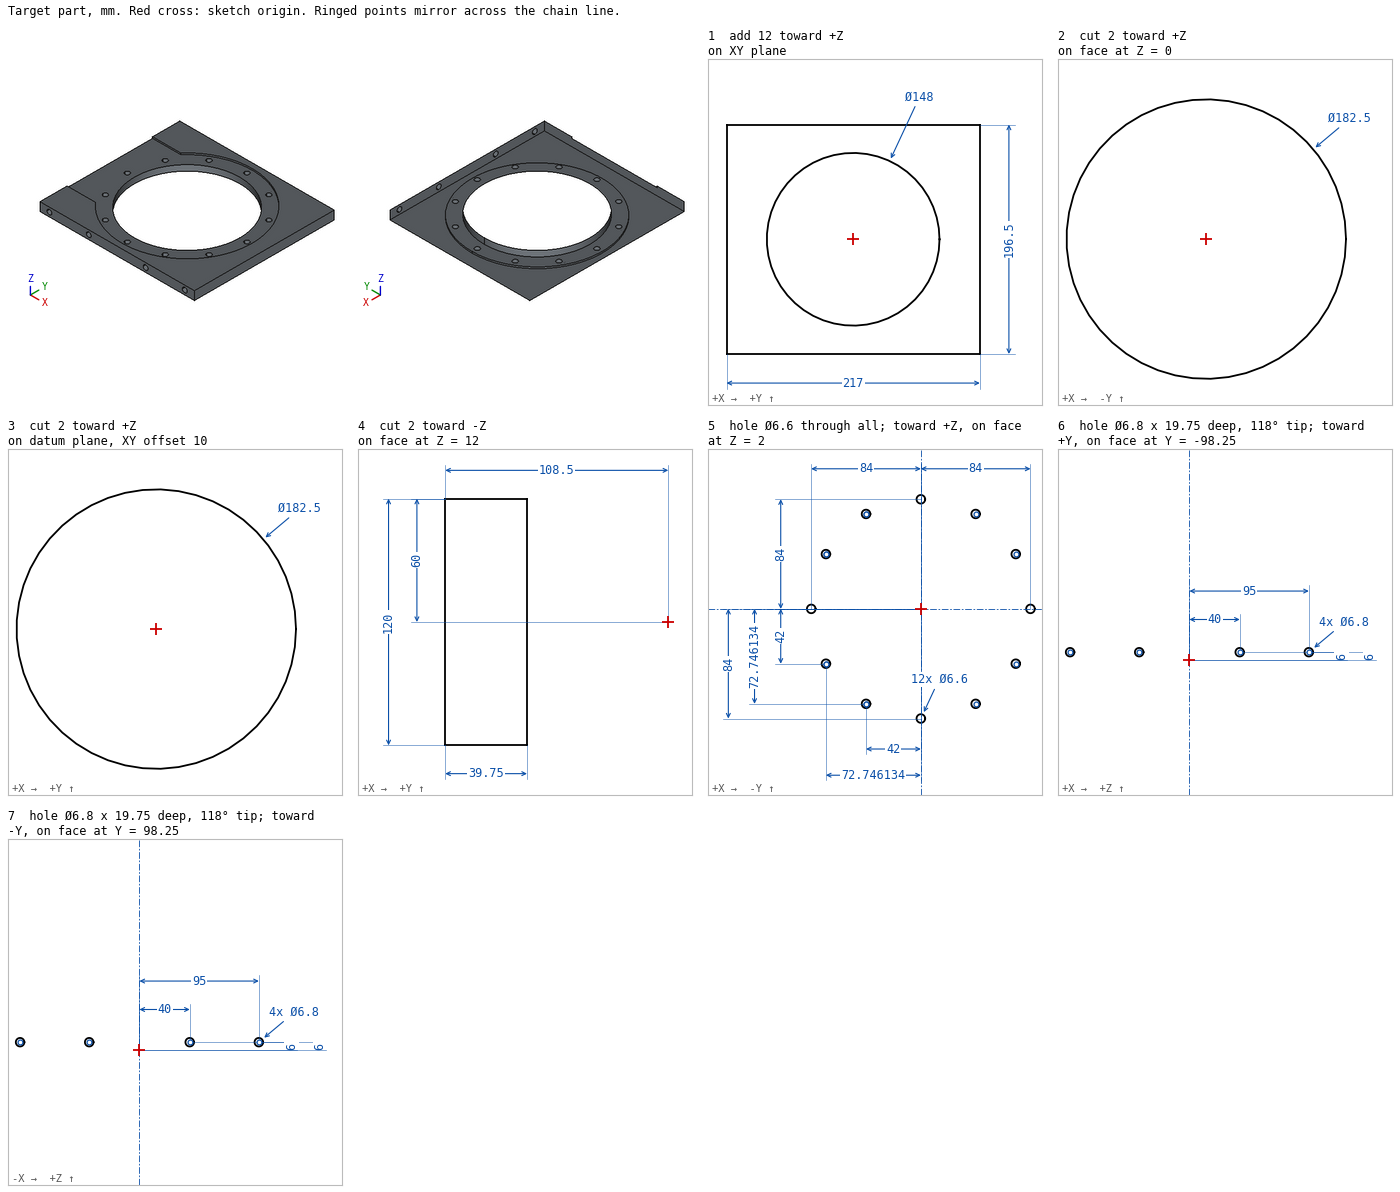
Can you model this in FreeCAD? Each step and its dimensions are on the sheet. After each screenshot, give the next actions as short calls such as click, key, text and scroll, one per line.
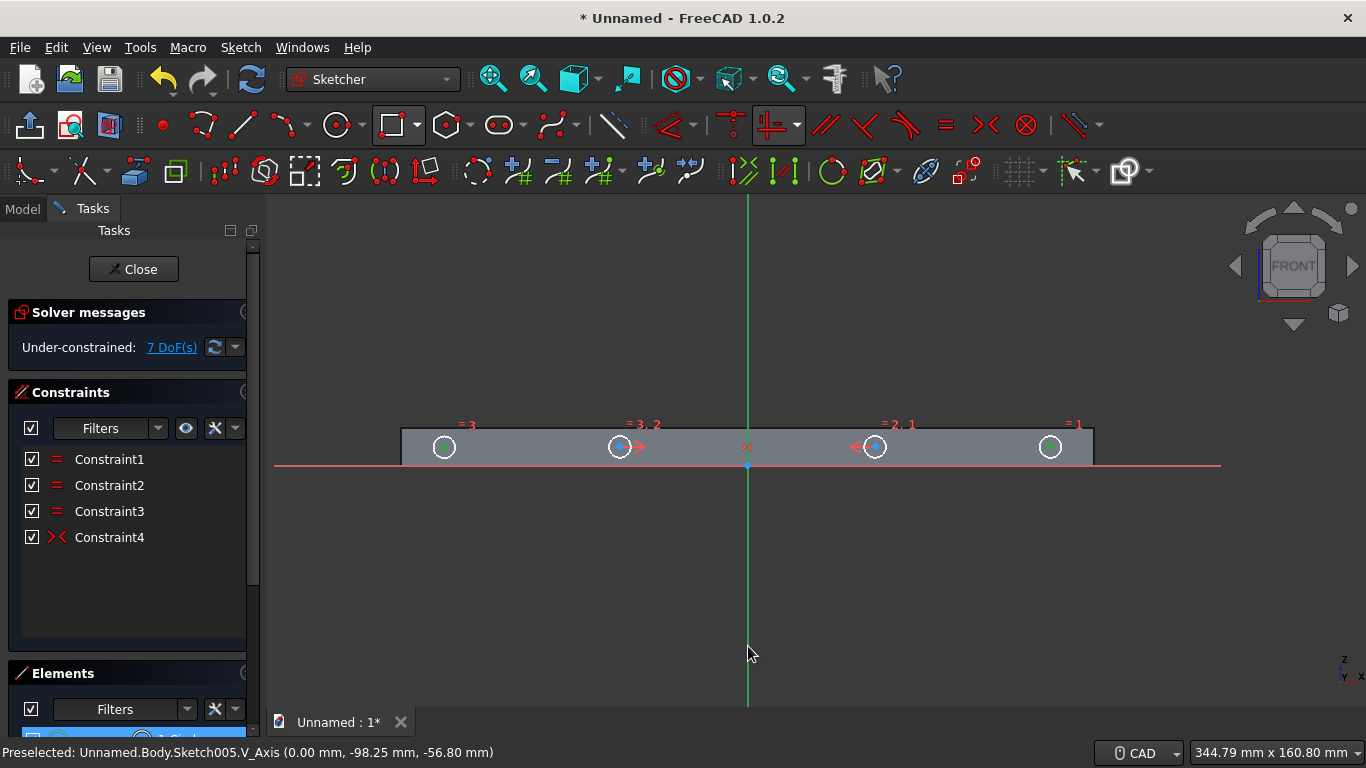
click(986, 126)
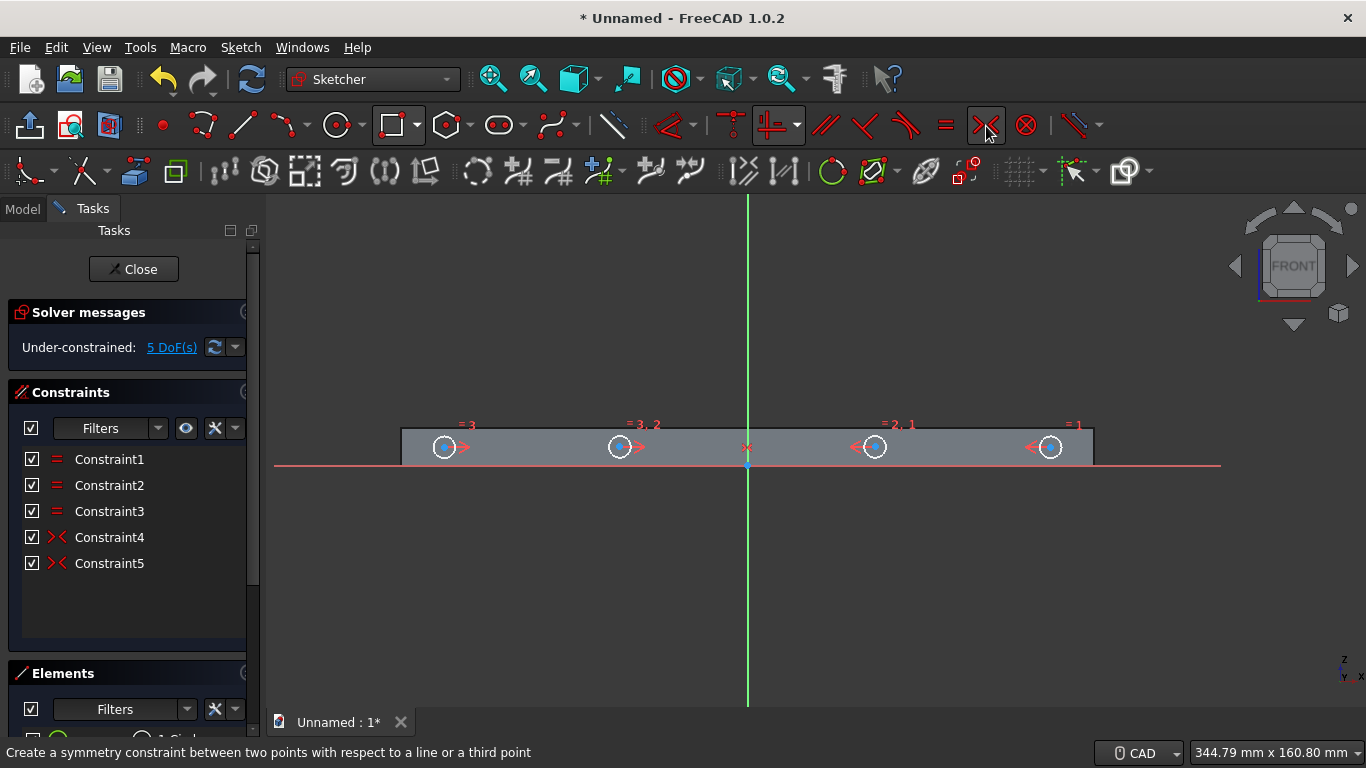
click(668, 126)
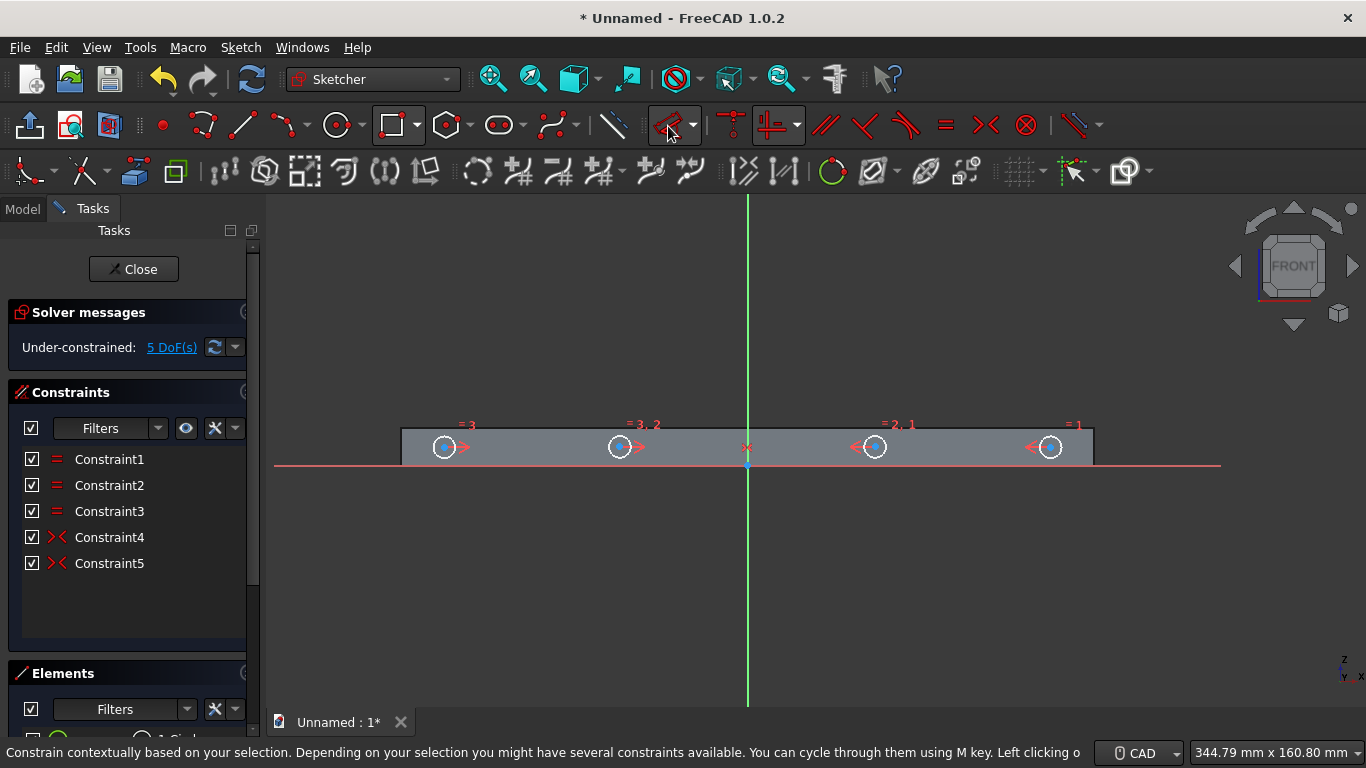
scroll(1058, 440, up, 4)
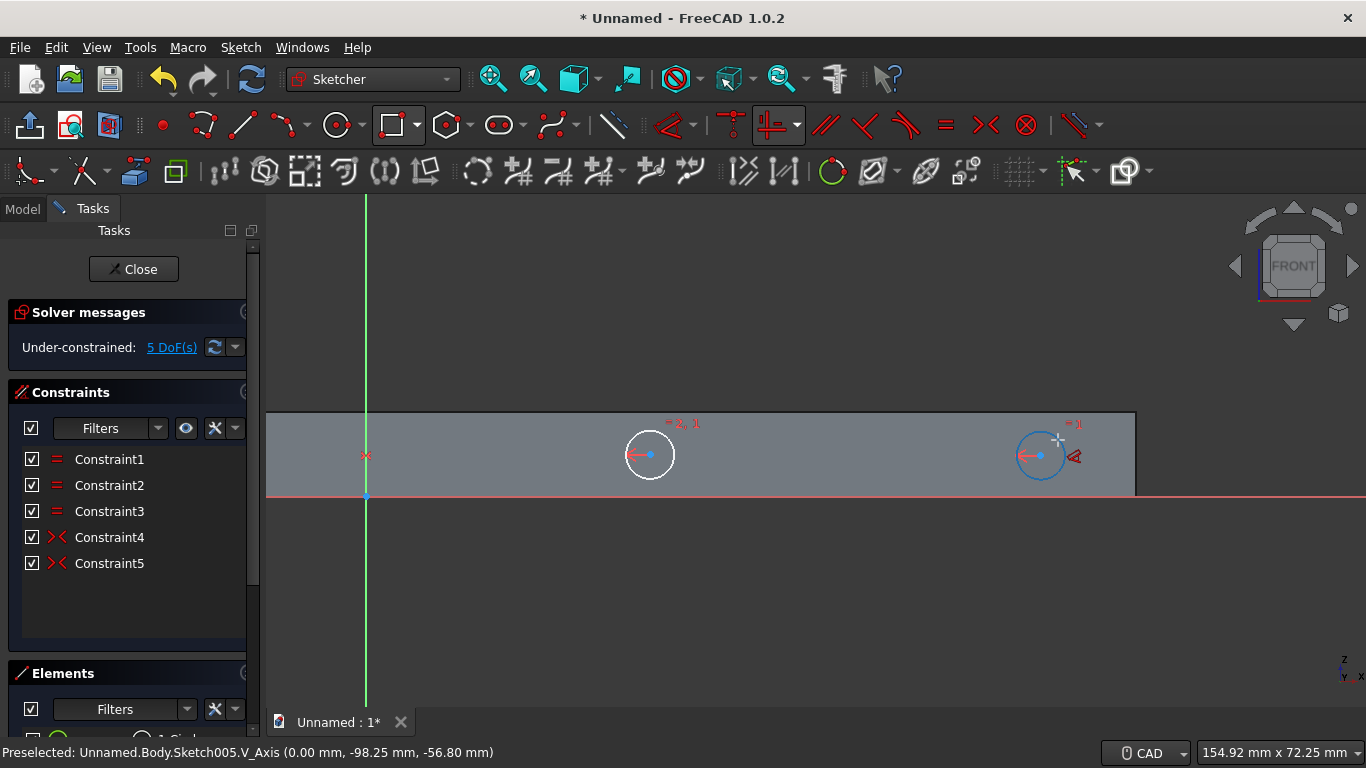
click(1058, 439)
click(1081, 417)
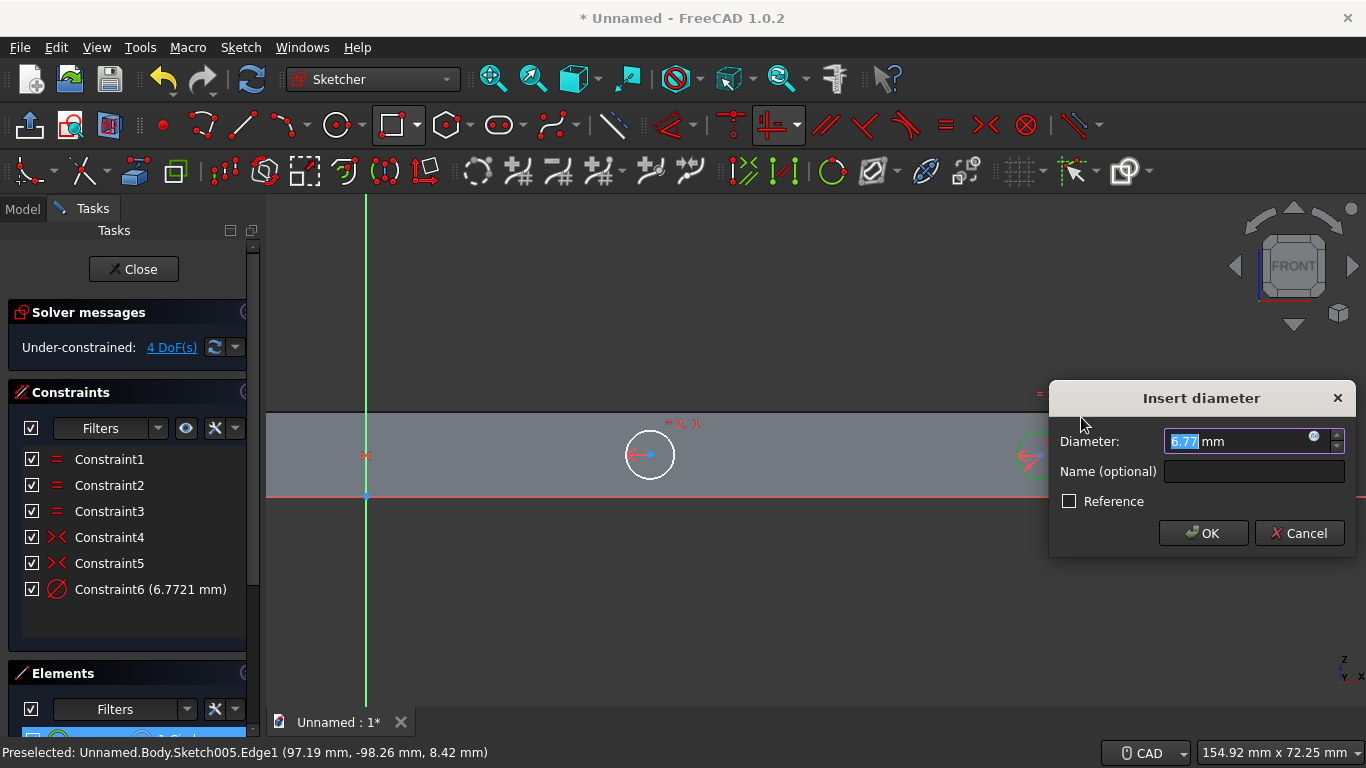
text(6.8)
key(Return)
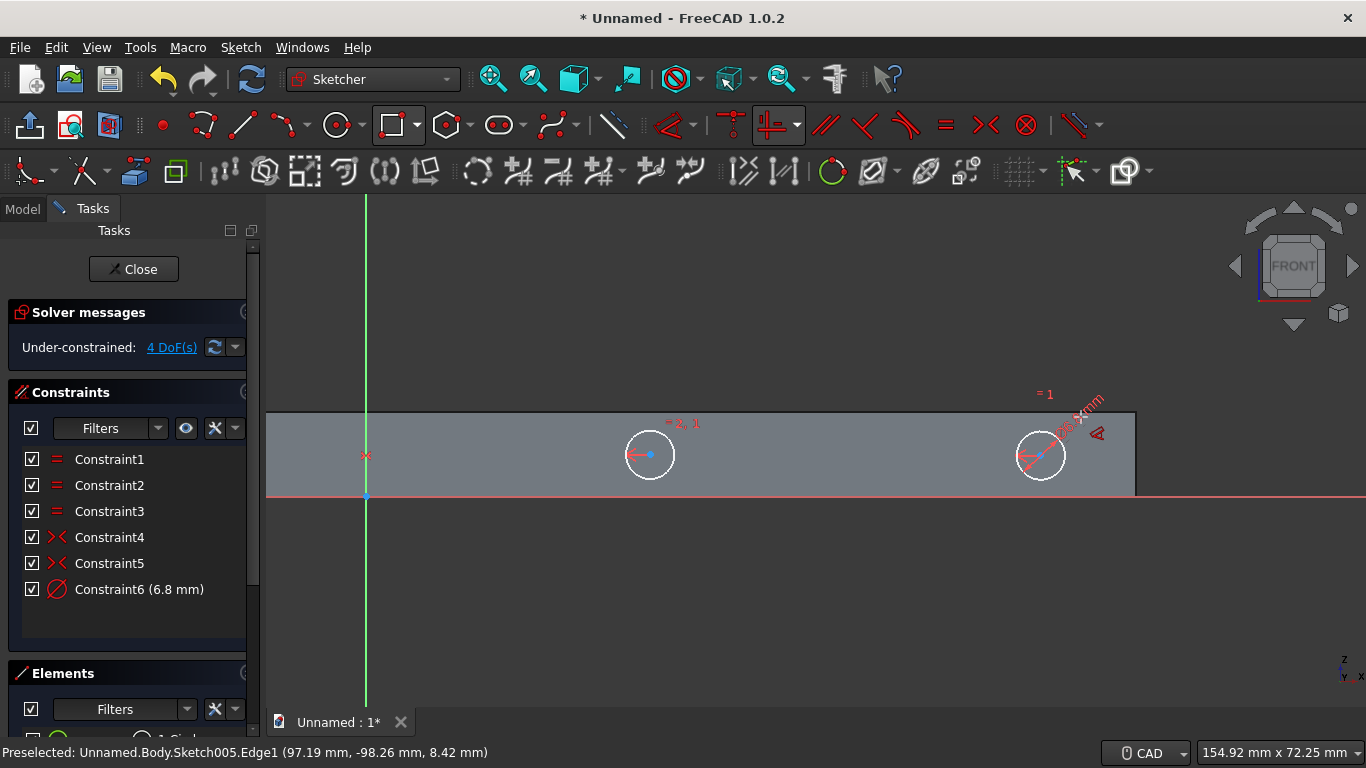
click(1041, 456)
click(1075, 476)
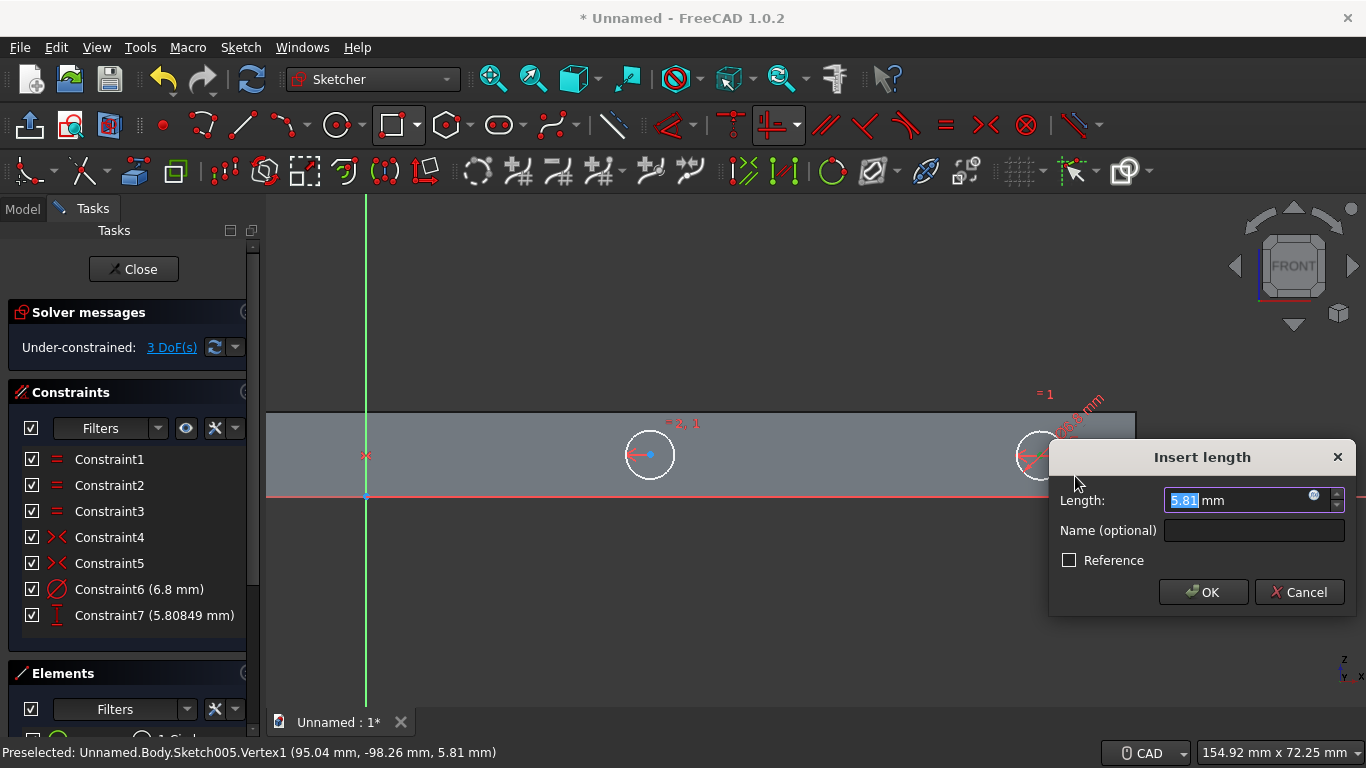
text(6)
key(Return)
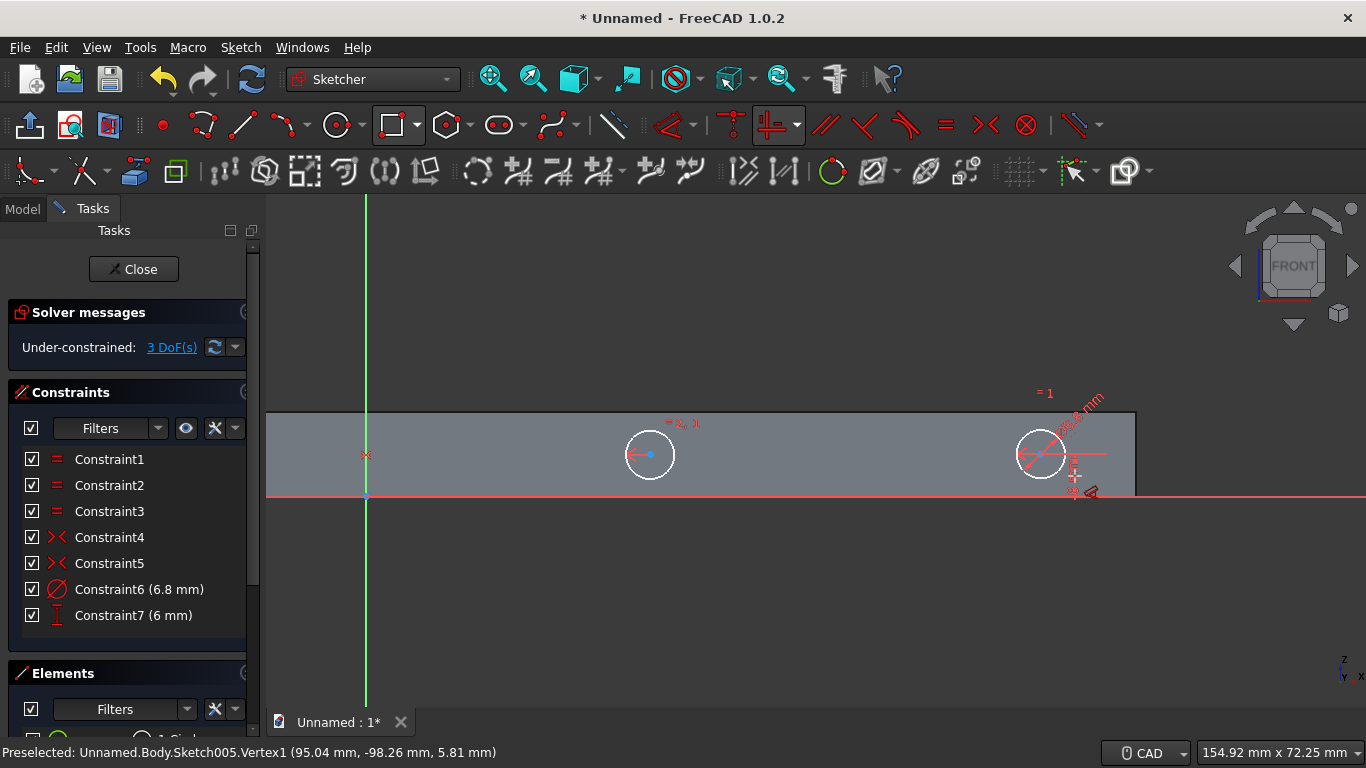
click(650, 455)
click(684, 476)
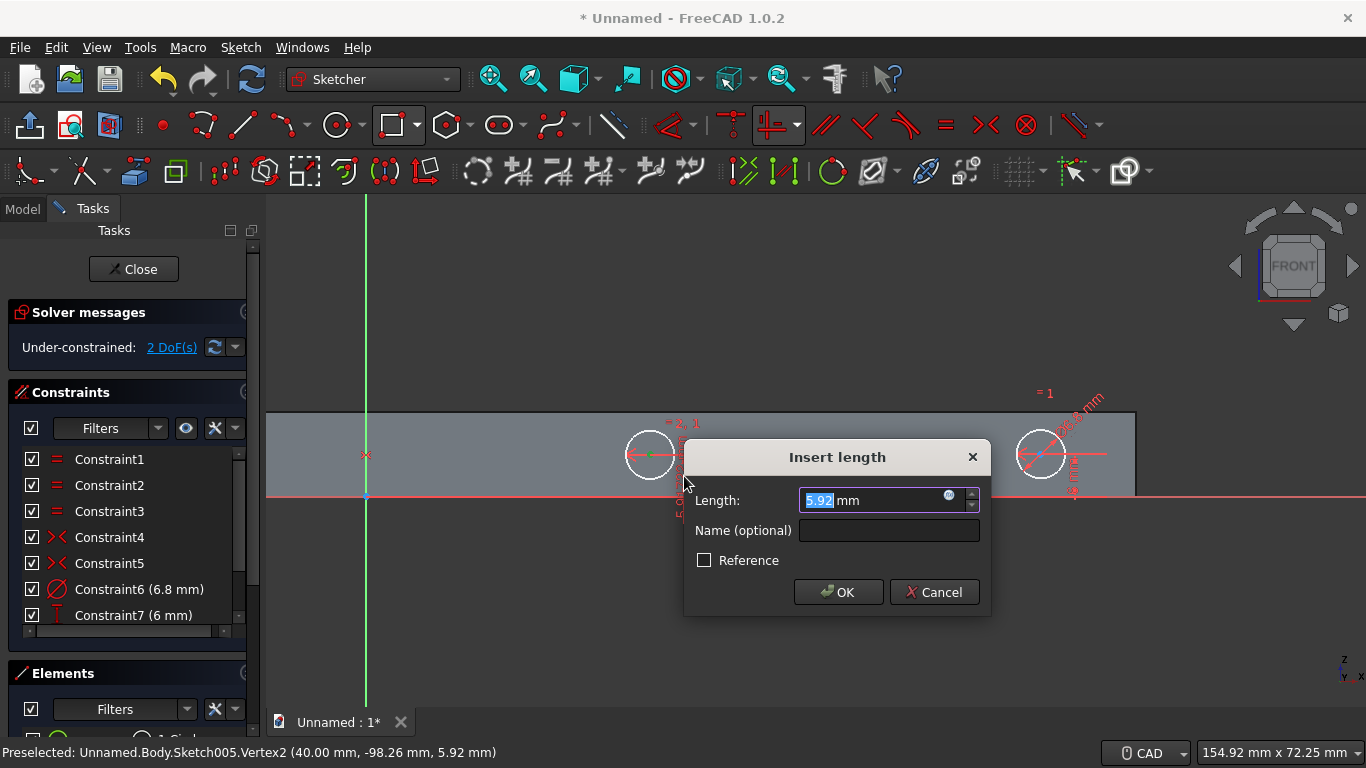
text(6)
key(Return)